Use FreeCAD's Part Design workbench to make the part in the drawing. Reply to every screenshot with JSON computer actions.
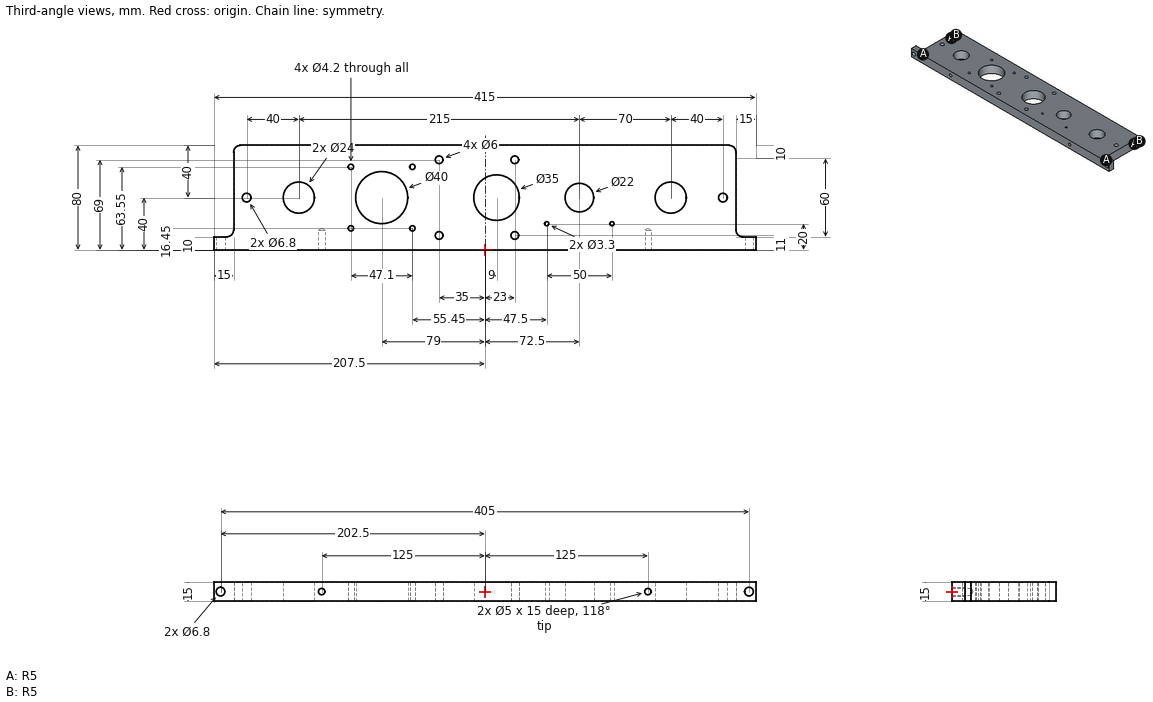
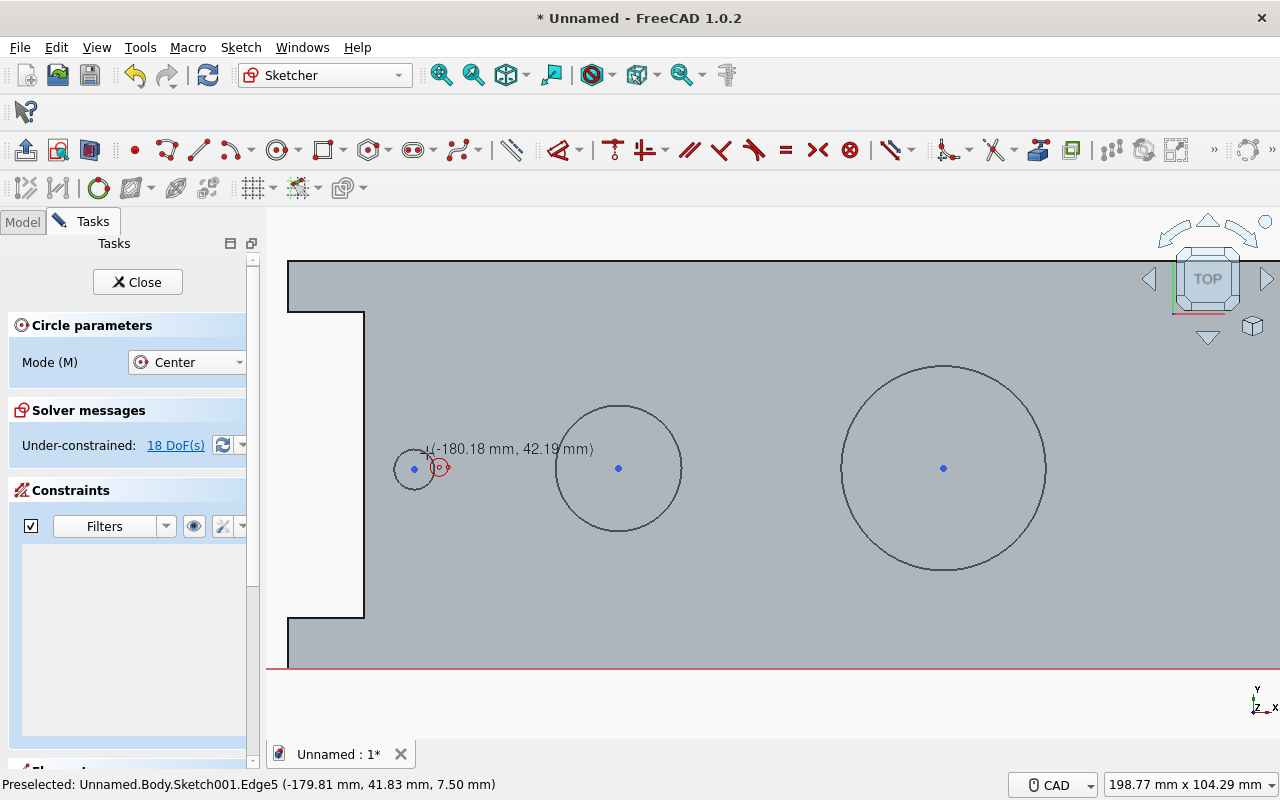
{"action": "scroll", "coordinate": [428, 454], "scroll_direction": "down", "scroll_amount": 6}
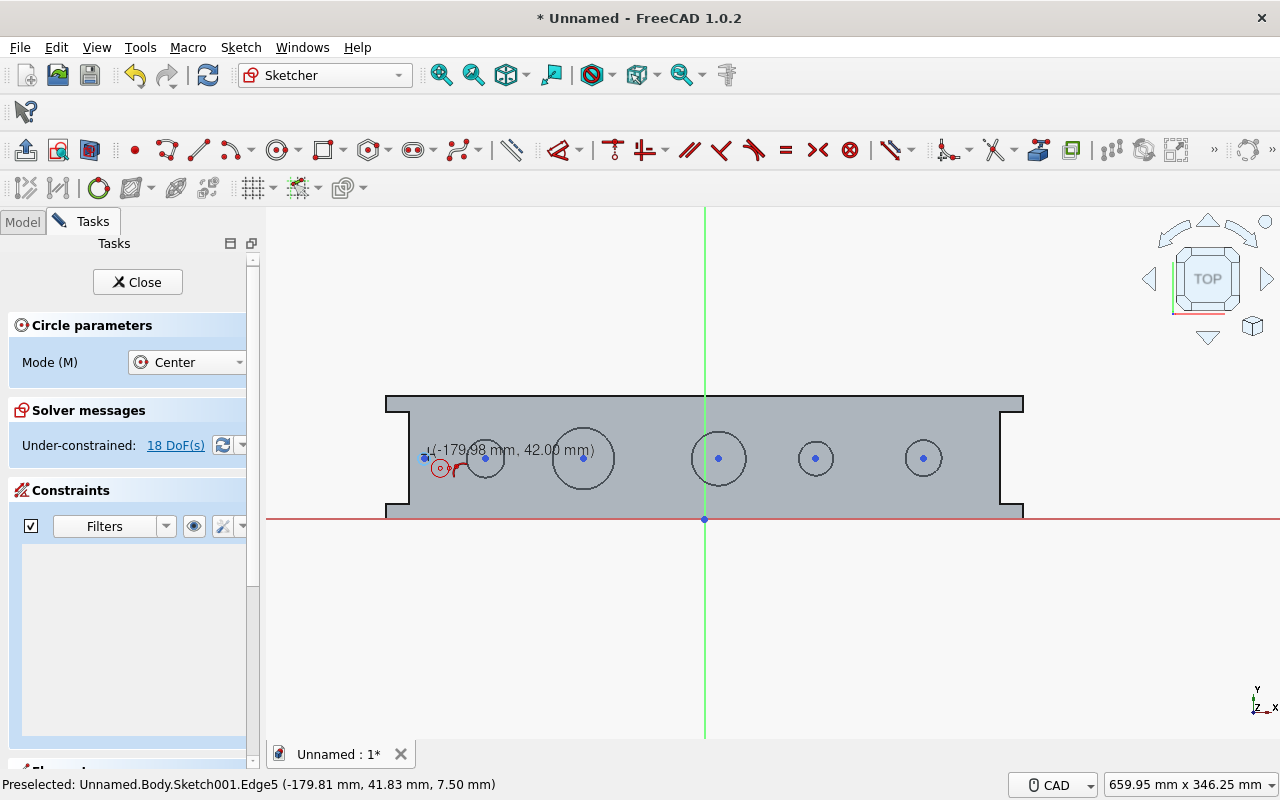
{"action": "scroll", "coordinate": [985, 458], "scroll_direction": "up", "scroll_amount": 8}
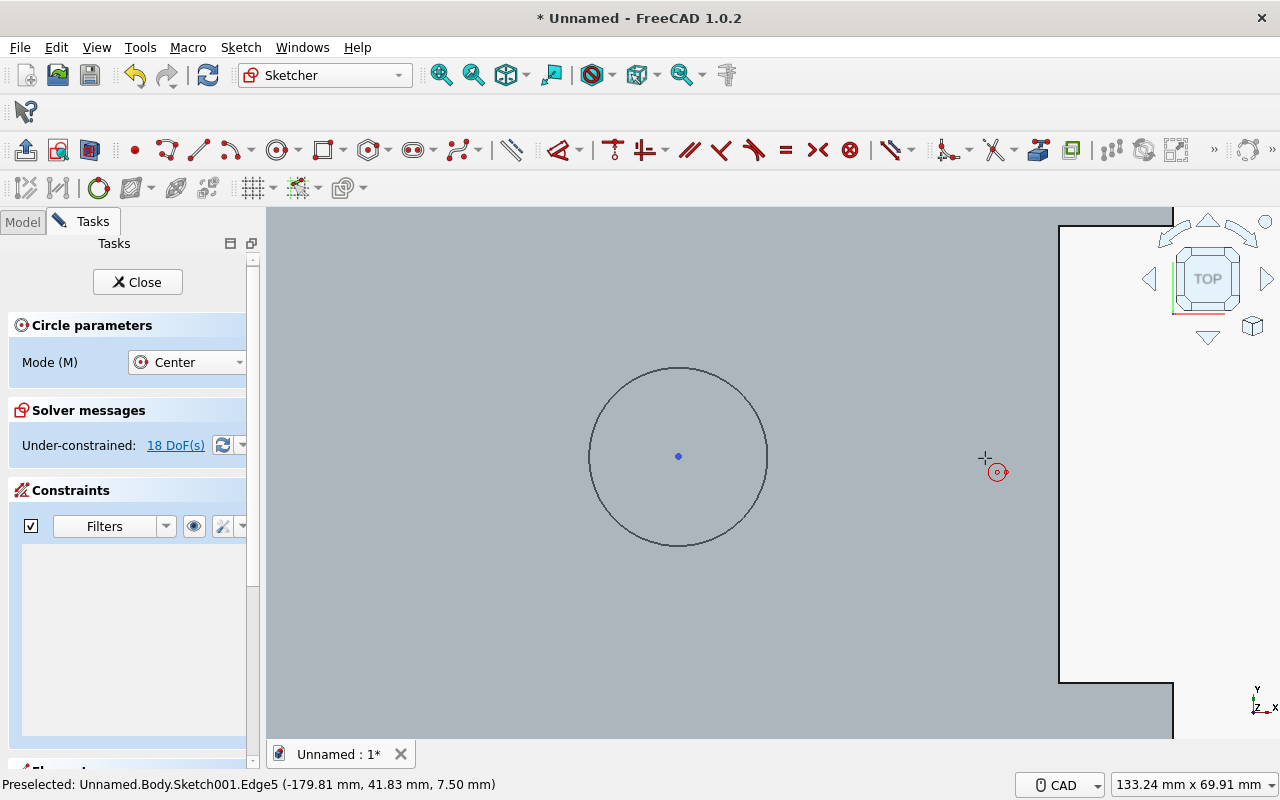
{"action": "scroll", "coordinate": [986, 458], "scroll_direction": "down", "scroll_amount": 8}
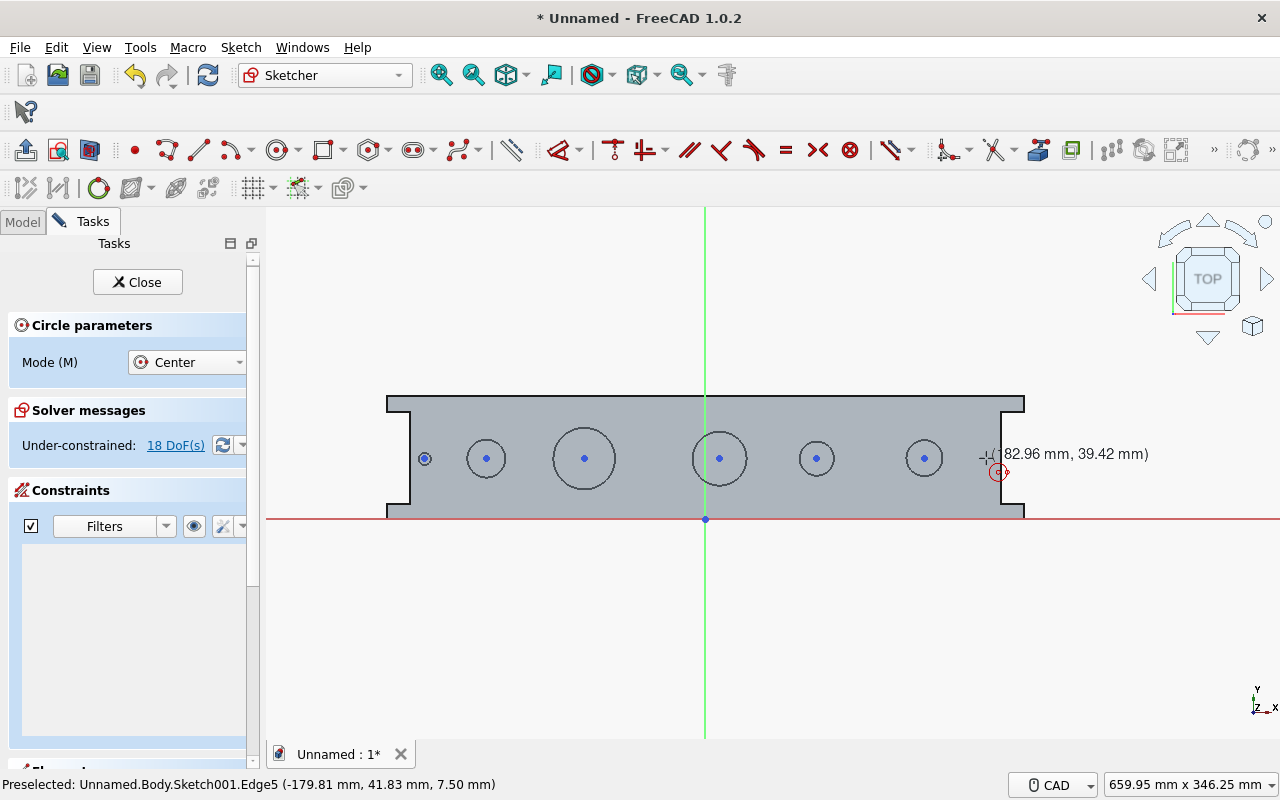
{"action": "left_click", "coordinate": [986, 458]}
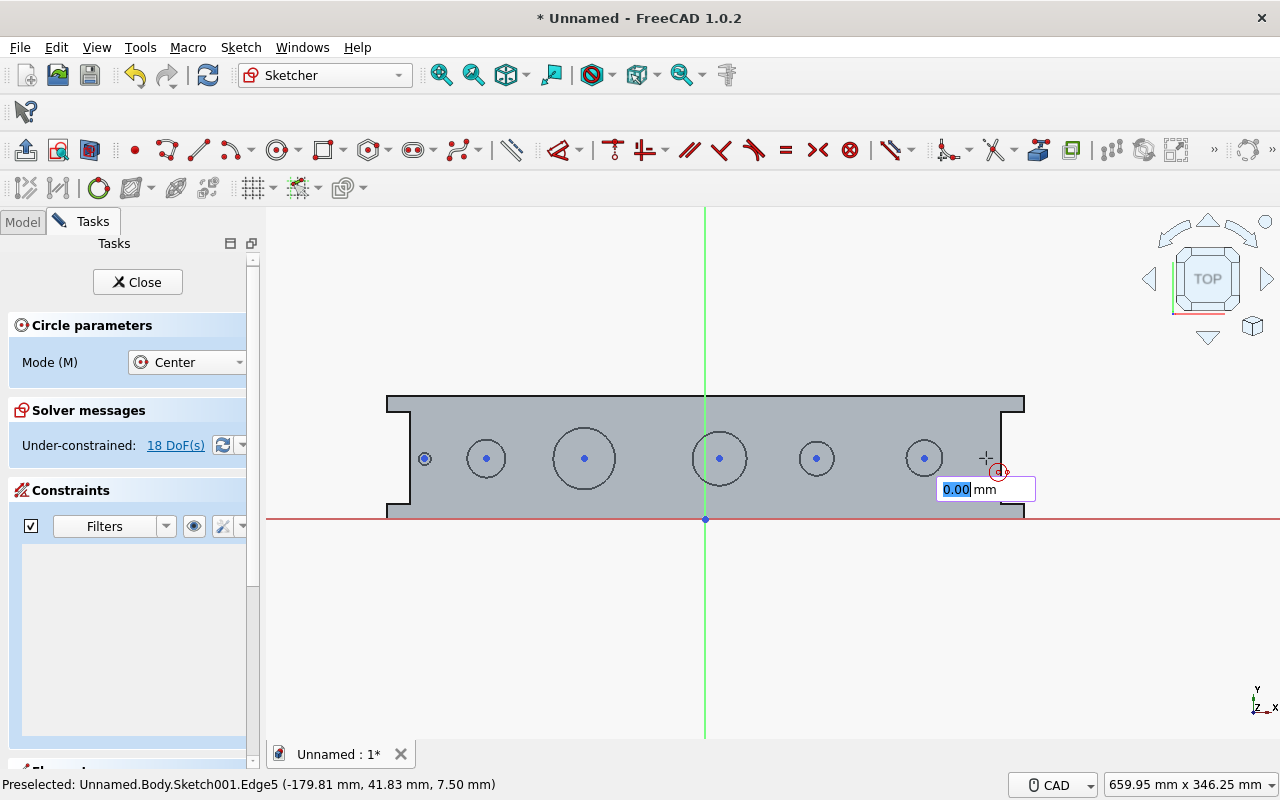
{"action": "scroll", "coordinate": [990, 454], "scroll_direction": "up", "scroll_amount": 6}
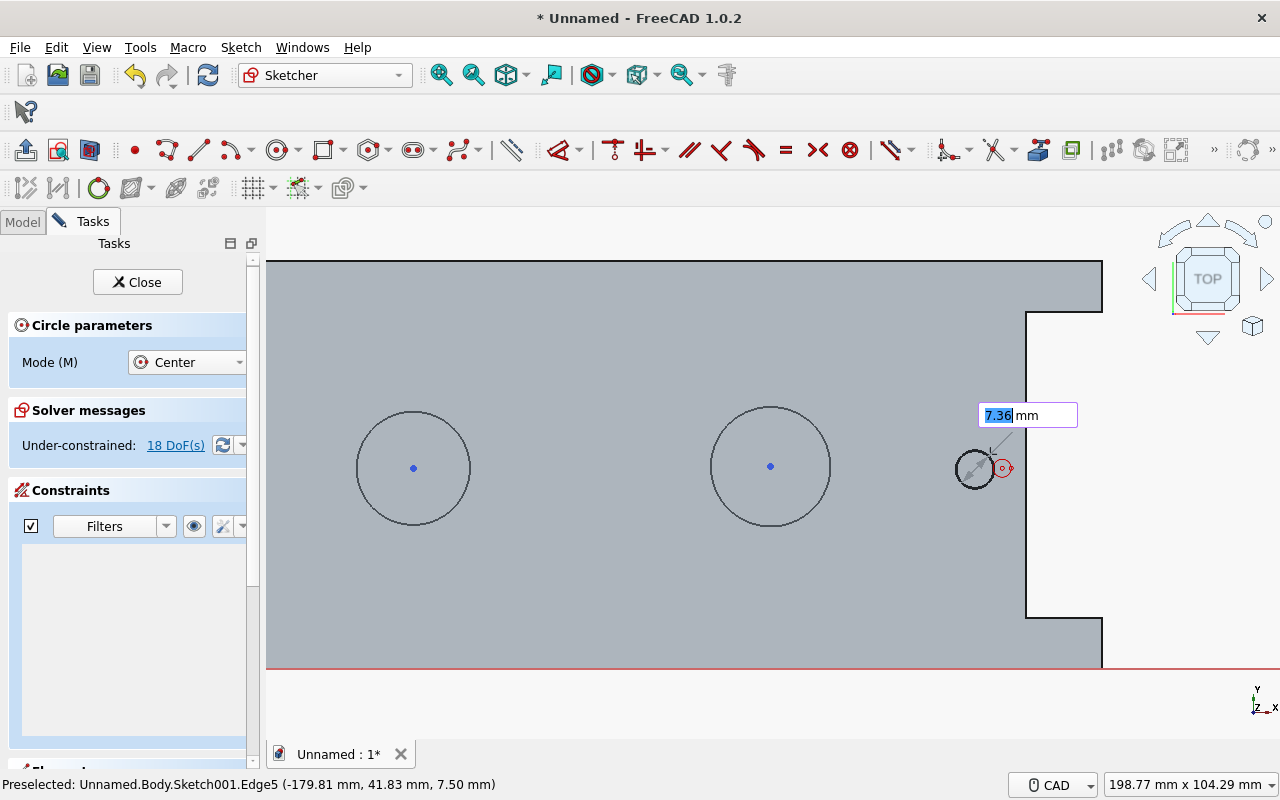
{"action": "left_click", "coordinate": [987, 453]}
{"action": "key", "text": "Escape"}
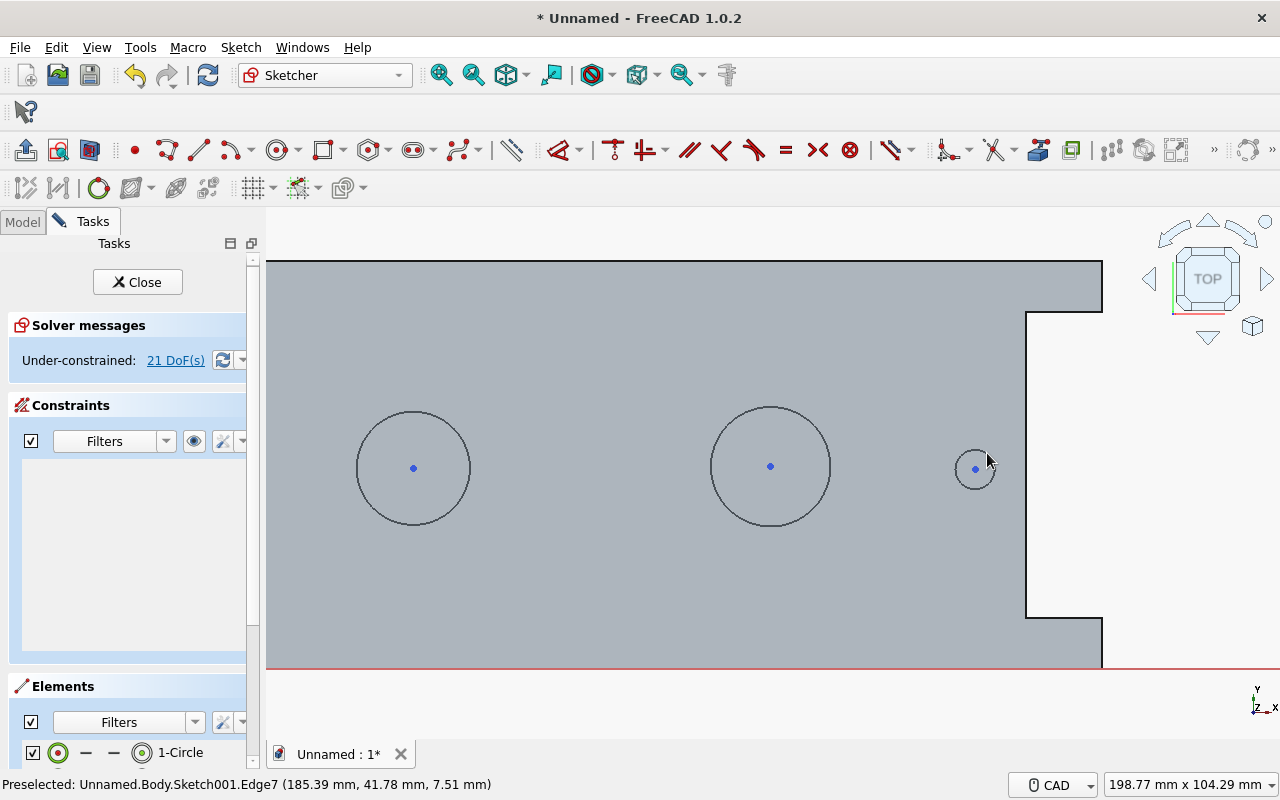
{"action": "scroll", "coordinate": [989, 454], "scroll_direction": "down", "scroll_amount": 6}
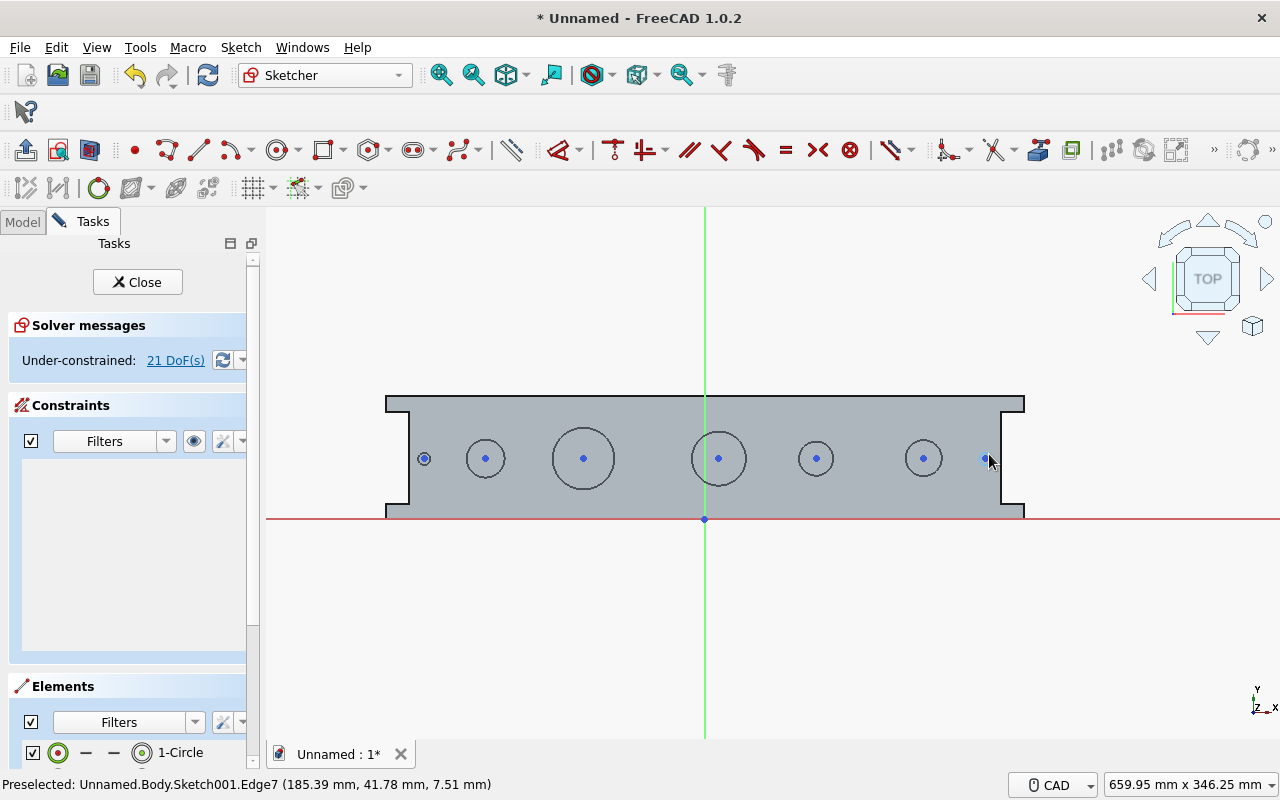
{"action": "left_click", "coordinate": [499, 445]}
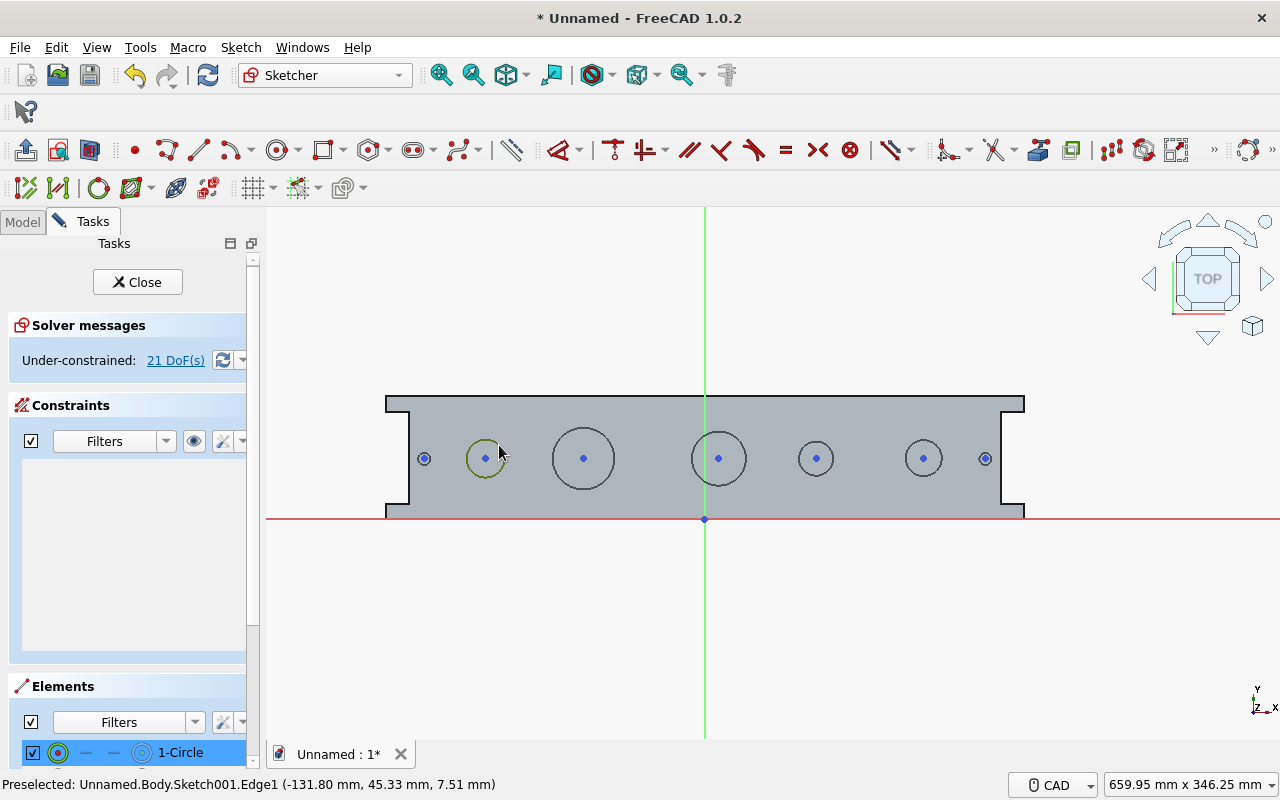
{"action": "left_click", "coordinate": [936, 445]}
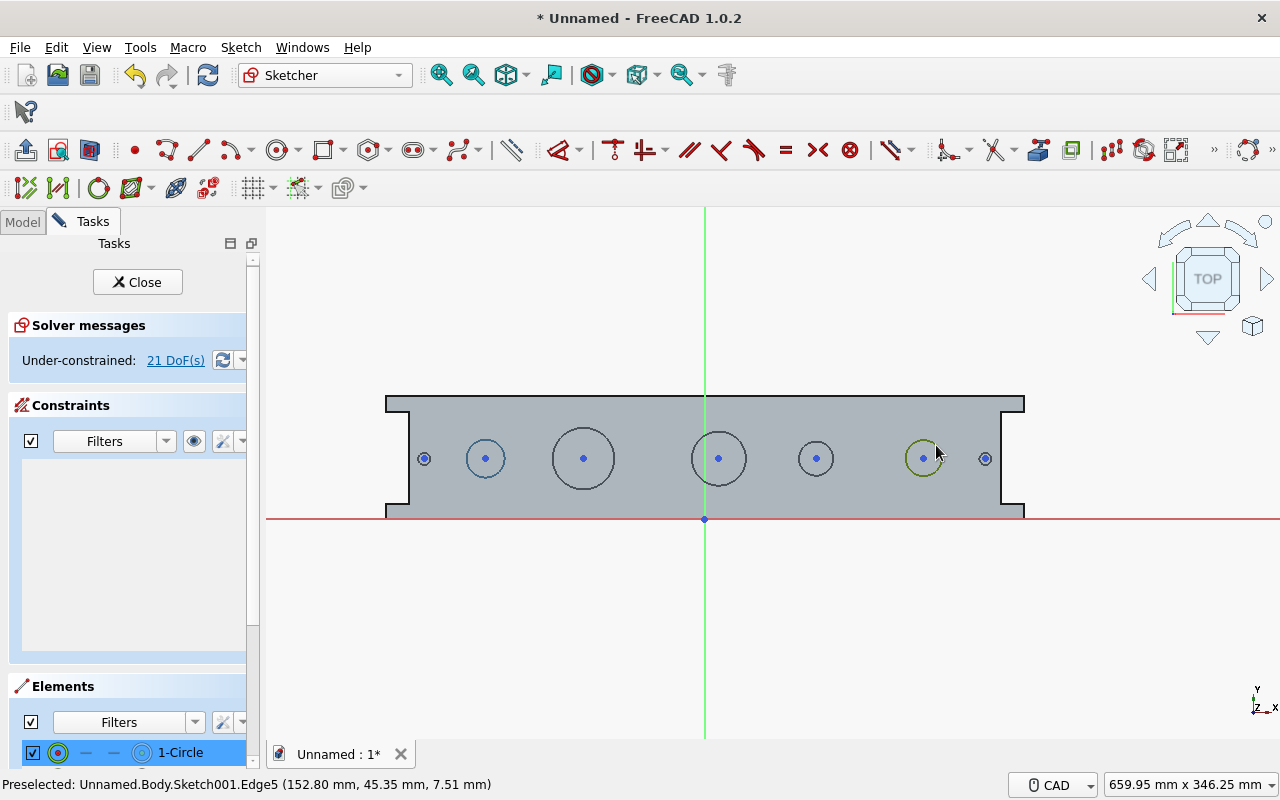
{"action": "left_click", "coordinate": [786, 150]}